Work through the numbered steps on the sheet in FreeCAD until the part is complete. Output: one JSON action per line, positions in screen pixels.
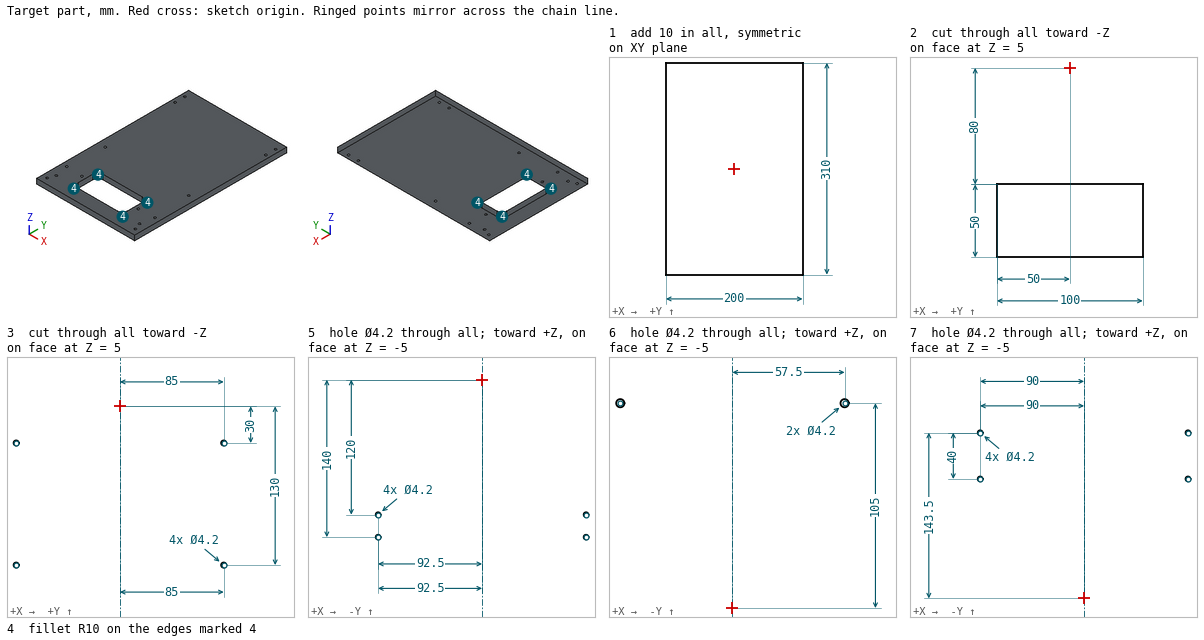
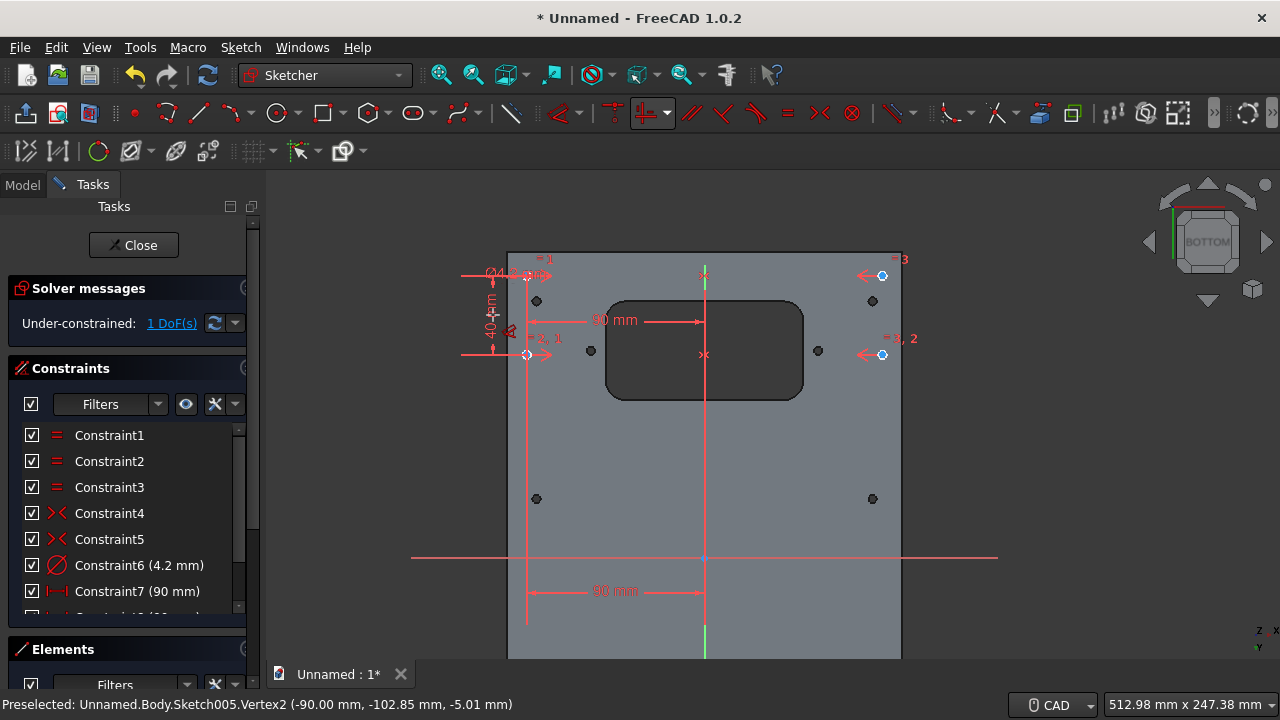
{"action": "left_click", "coordinate": [527, 276]}
{"action": "left_click", "coordinate": [493, 417]}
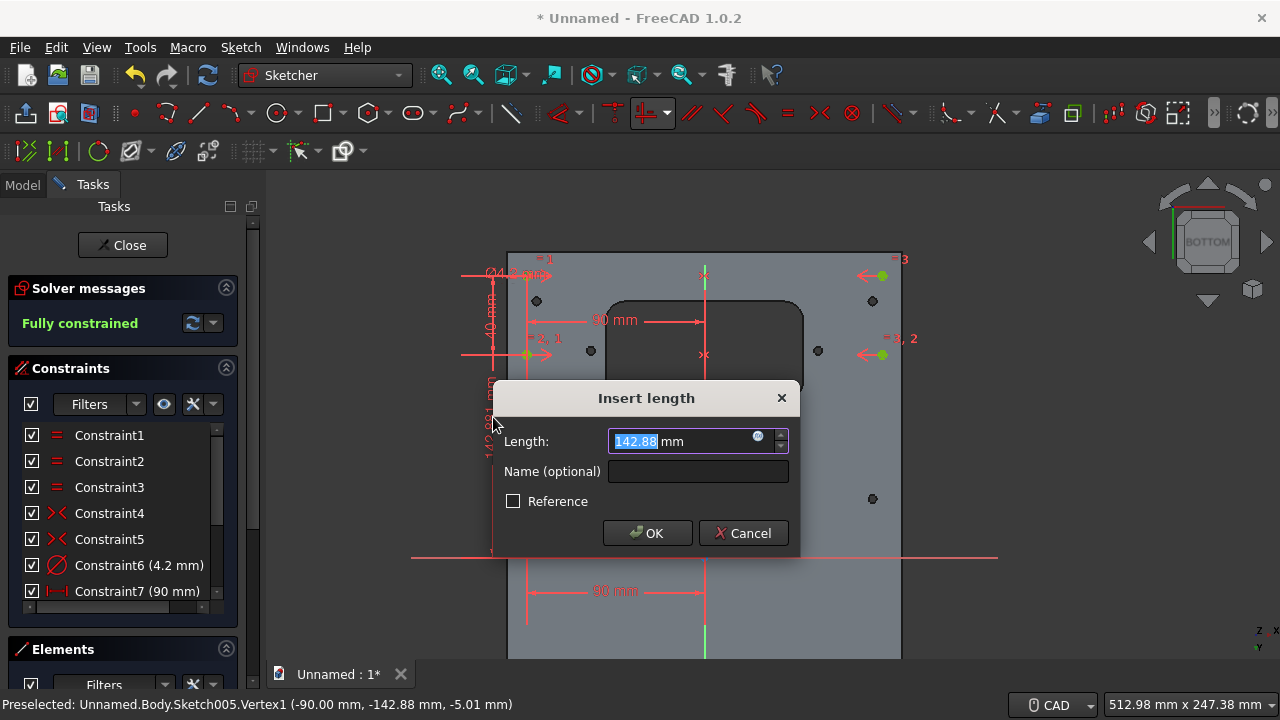
{"action": "type", "text": "143.5"}
{"action": "key", "text": "Return"}
{"action": "key", "text": "Escape"}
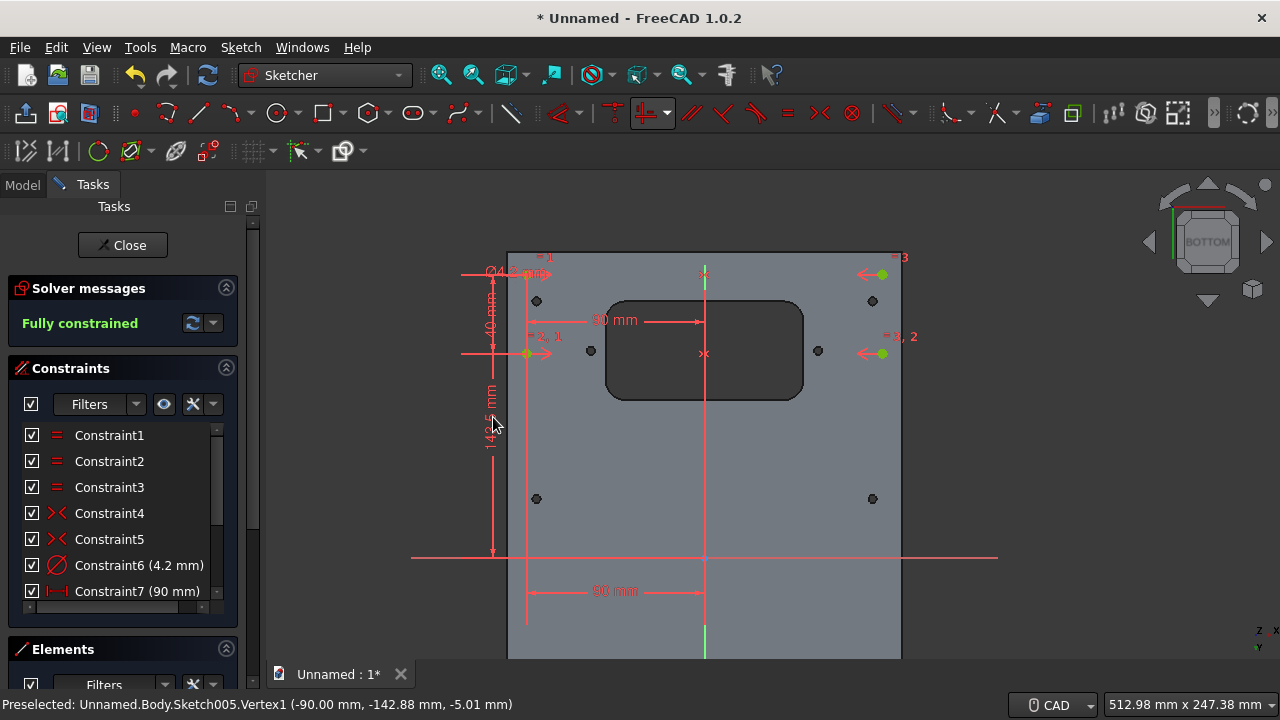
{"action": "left_click", "coordinate": [123, 245]}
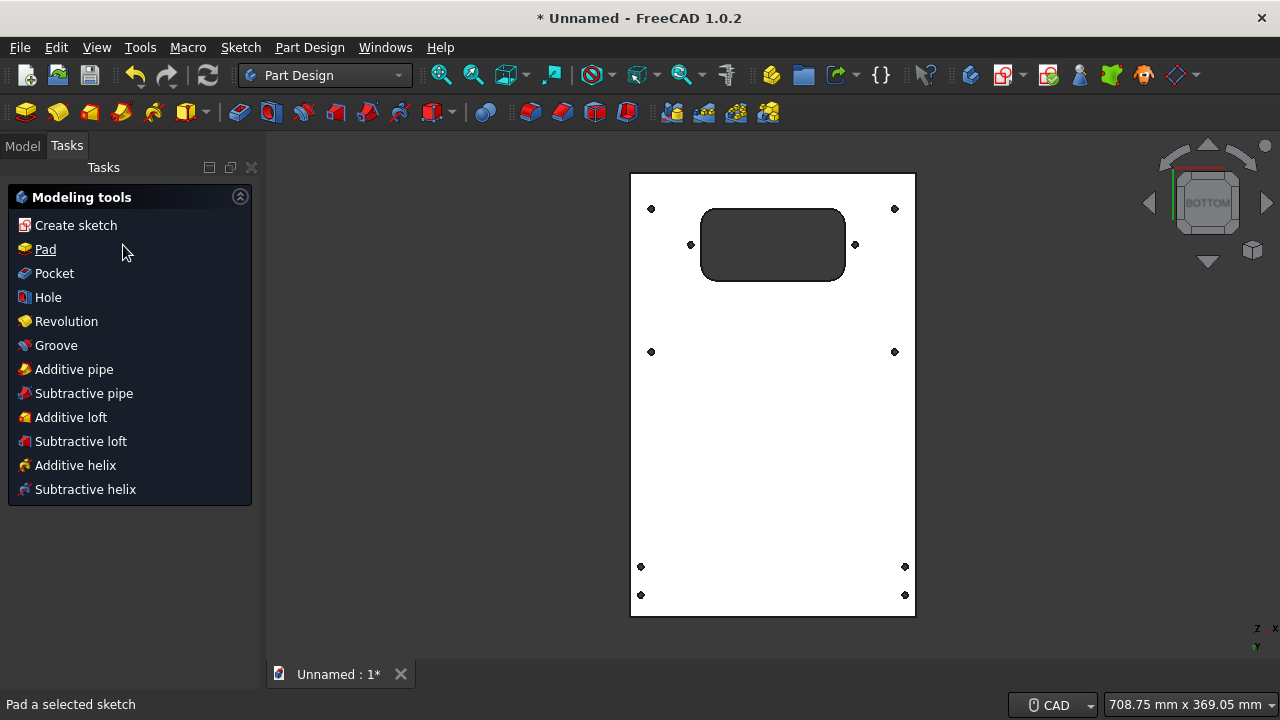
{"action": "left_click", "coordinate": [272, 112]}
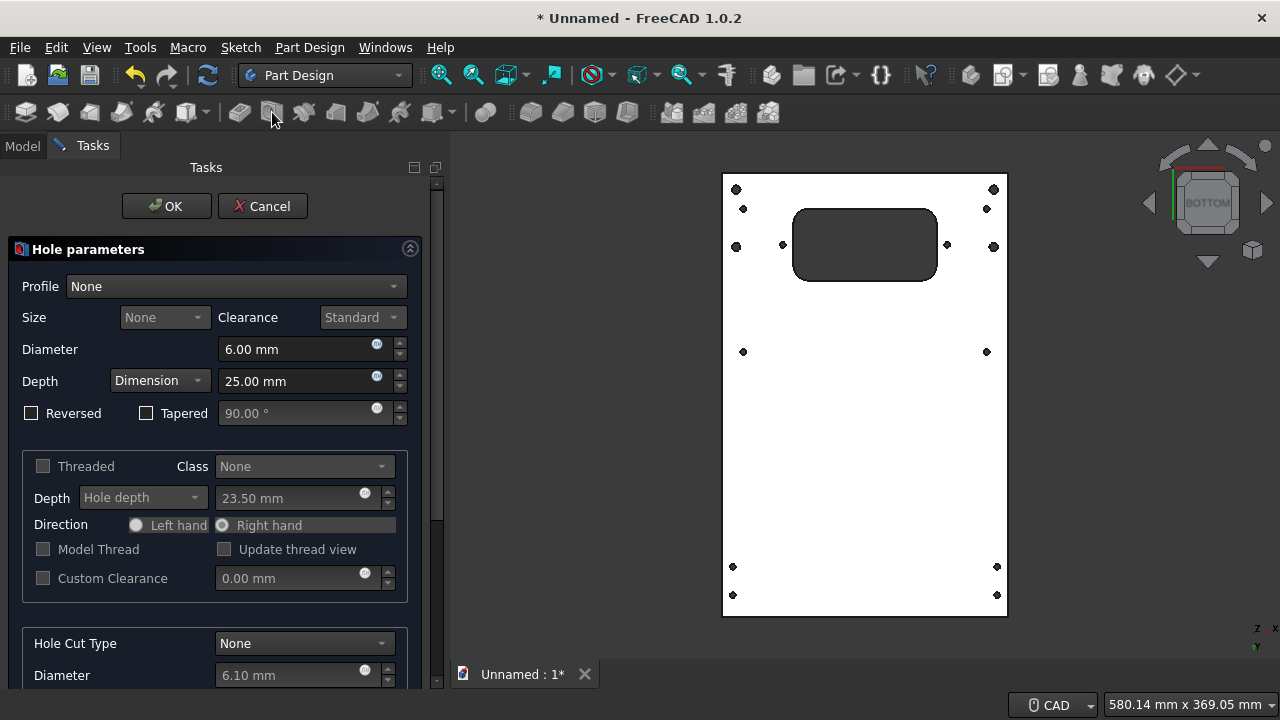
{"action": "triple_click", "coordinate": [305, 349]}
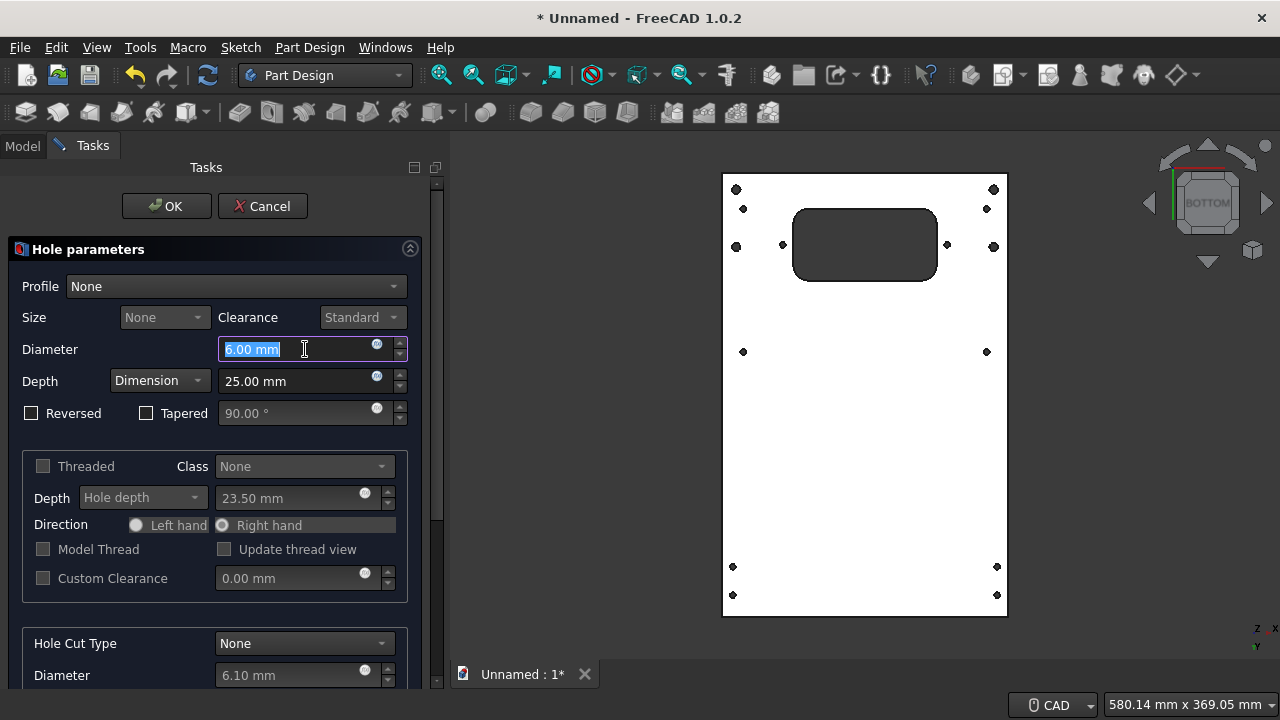
{"action": "type", "text": "4.2"}
{"action": "key", "text": "Tab"}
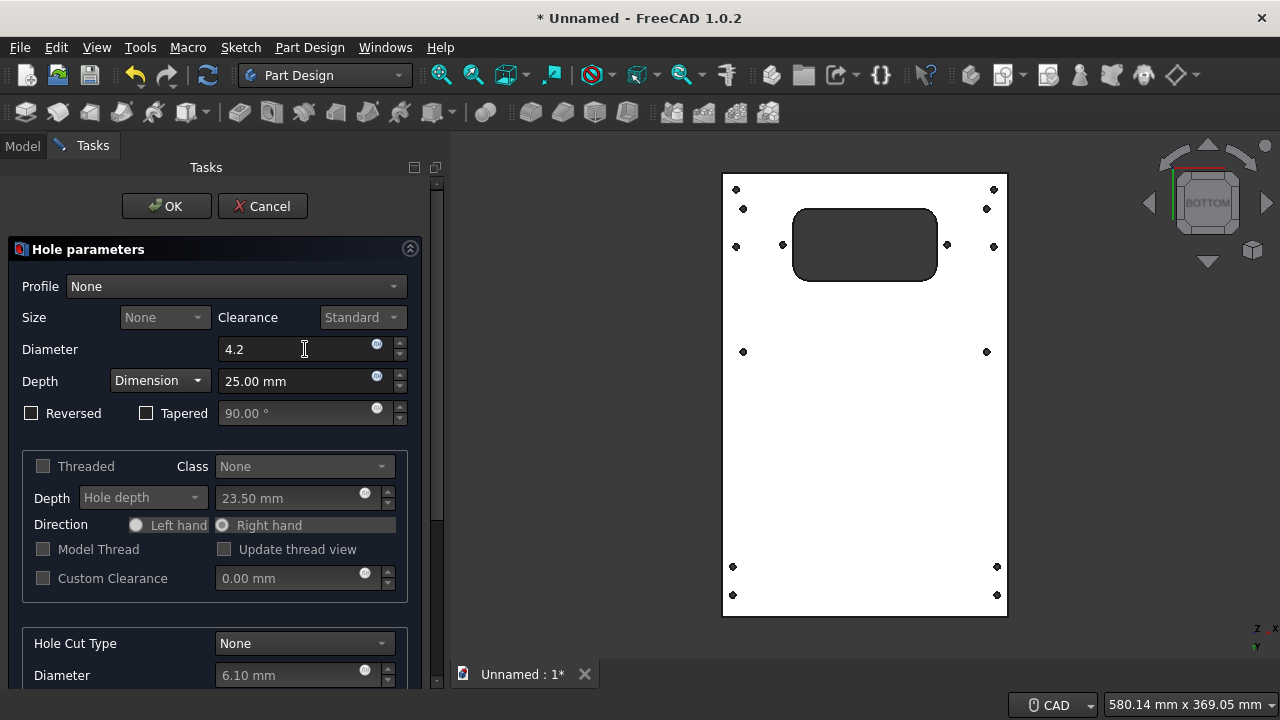
{"action": "left_click", "coordinate": [161, 380]}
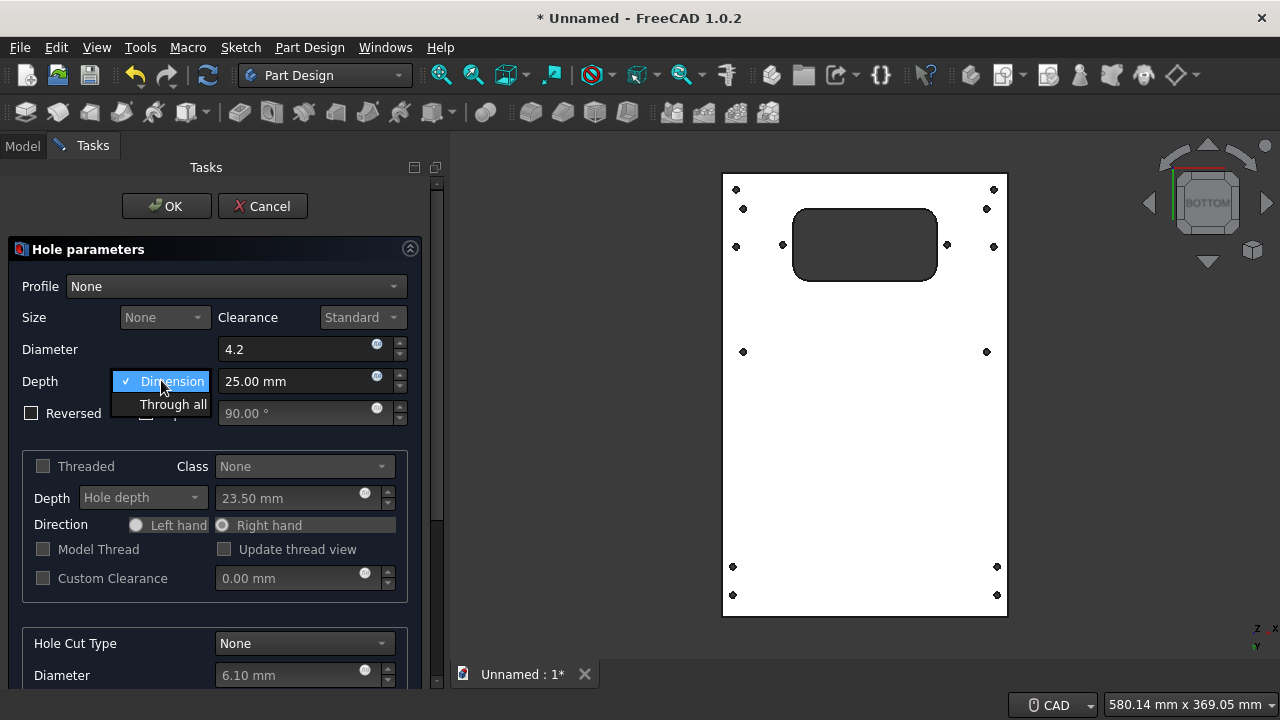
{"action": "left_click", "coordinate": [160, 404]}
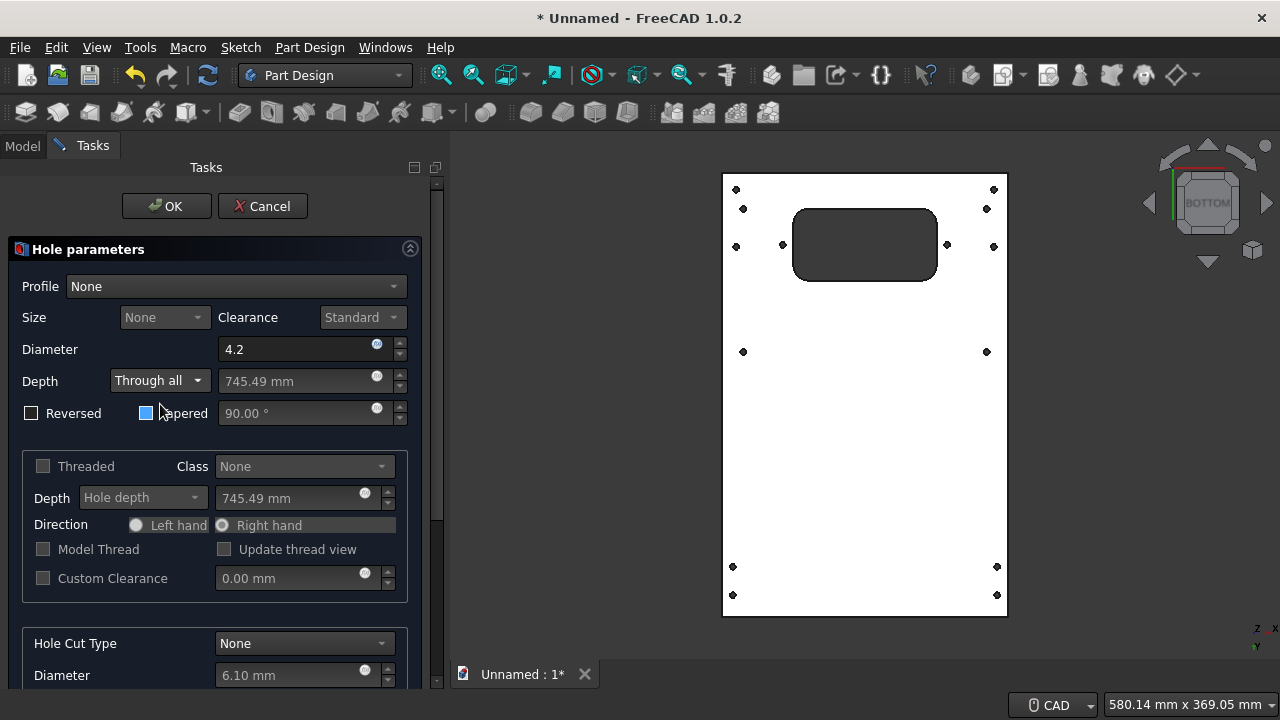
{"action": "left_click", "coordinate": [167, 206]}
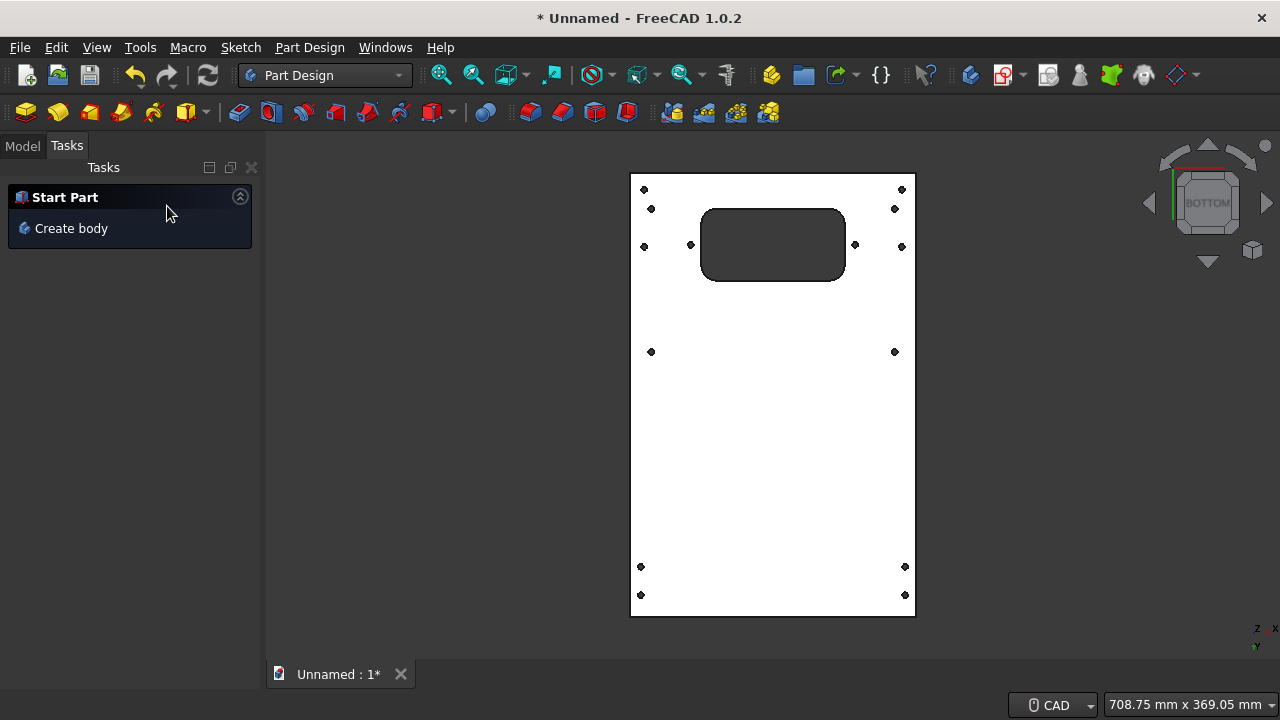
{"action": "key", "text": "0"}